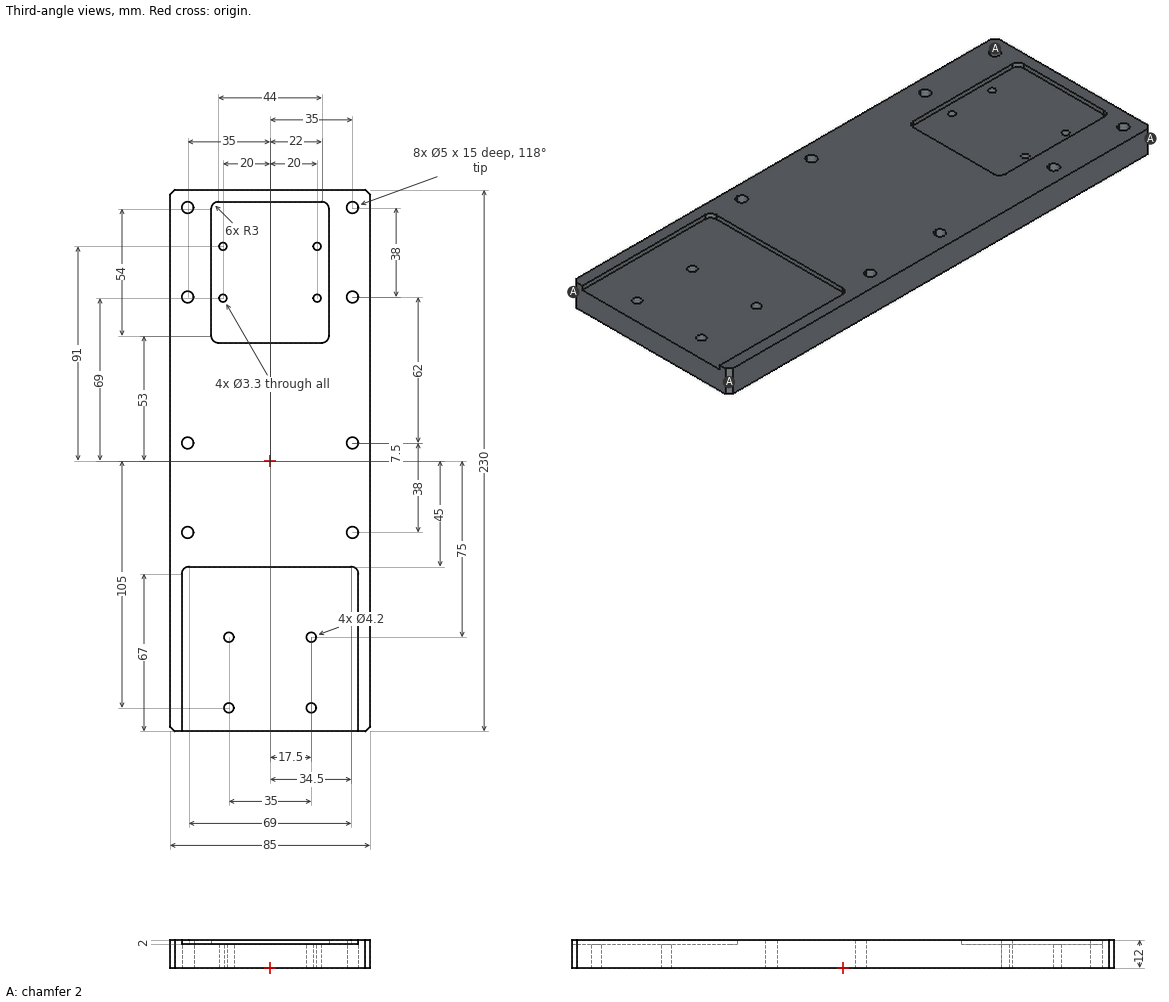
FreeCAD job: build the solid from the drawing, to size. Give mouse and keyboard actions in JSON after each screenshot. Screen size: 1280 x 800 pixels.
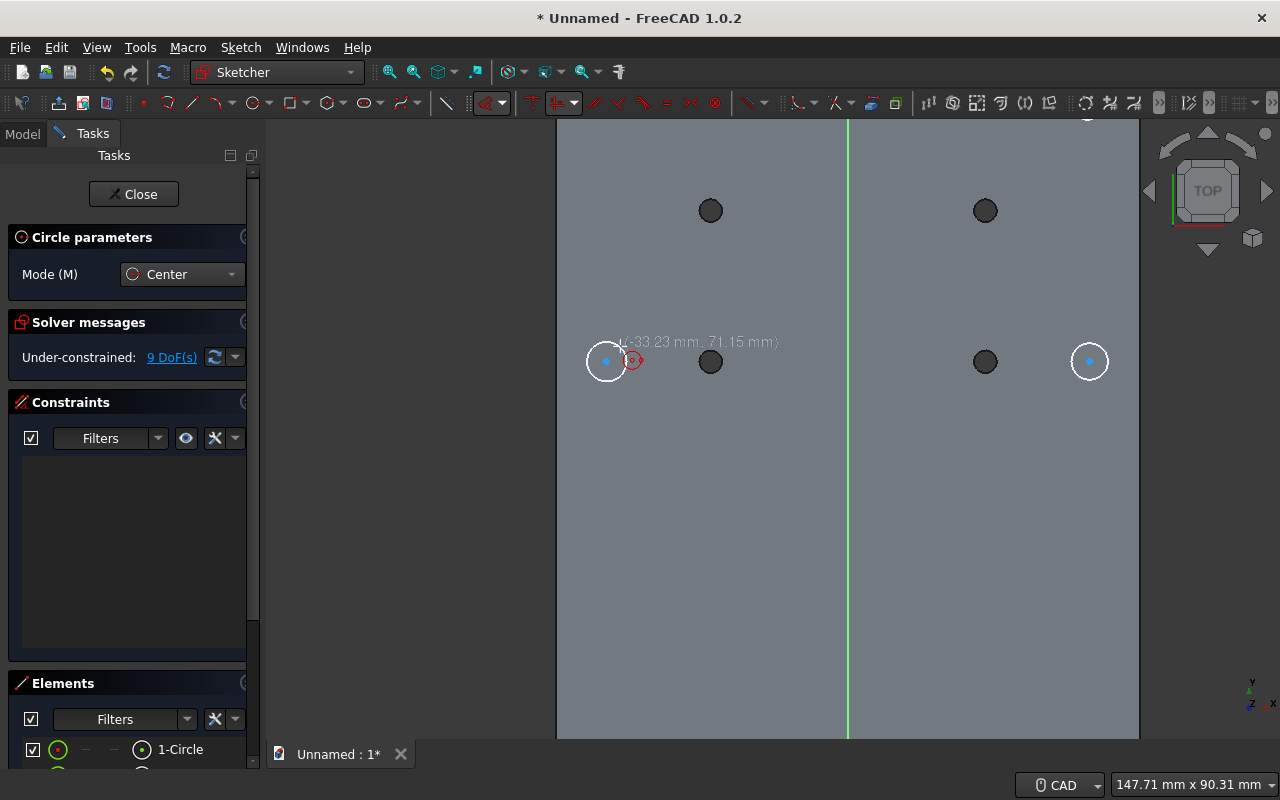
{"action": "scroll", "coordinate": [621, 346], "scroll_direction": "down", "scroll_amount": 5}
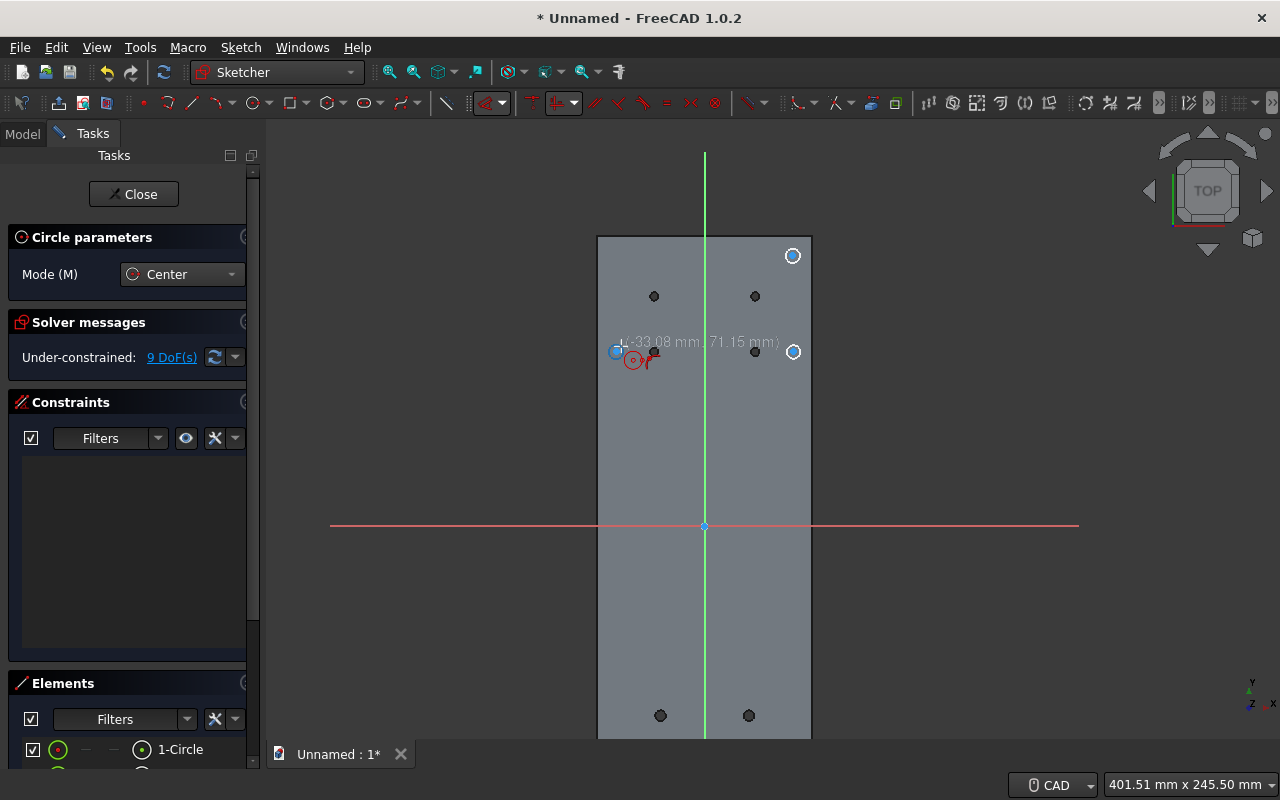
{"action": "scroll", "coordinate": [616, 255], "scroll_direction": "up", "scroll_amount": 7}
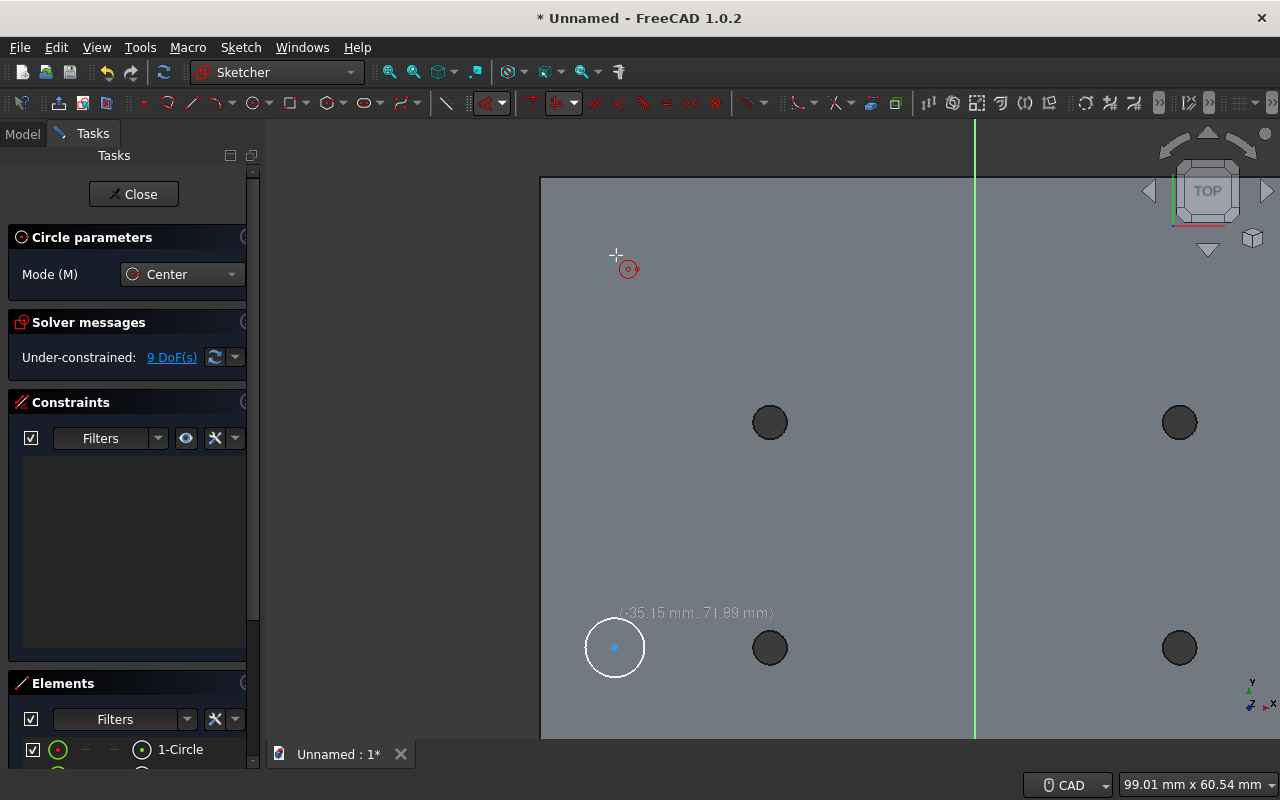
{"action": "scroll", "coordinate": [616, 255], "scroll_direction": "down", "scroll_amount": 7}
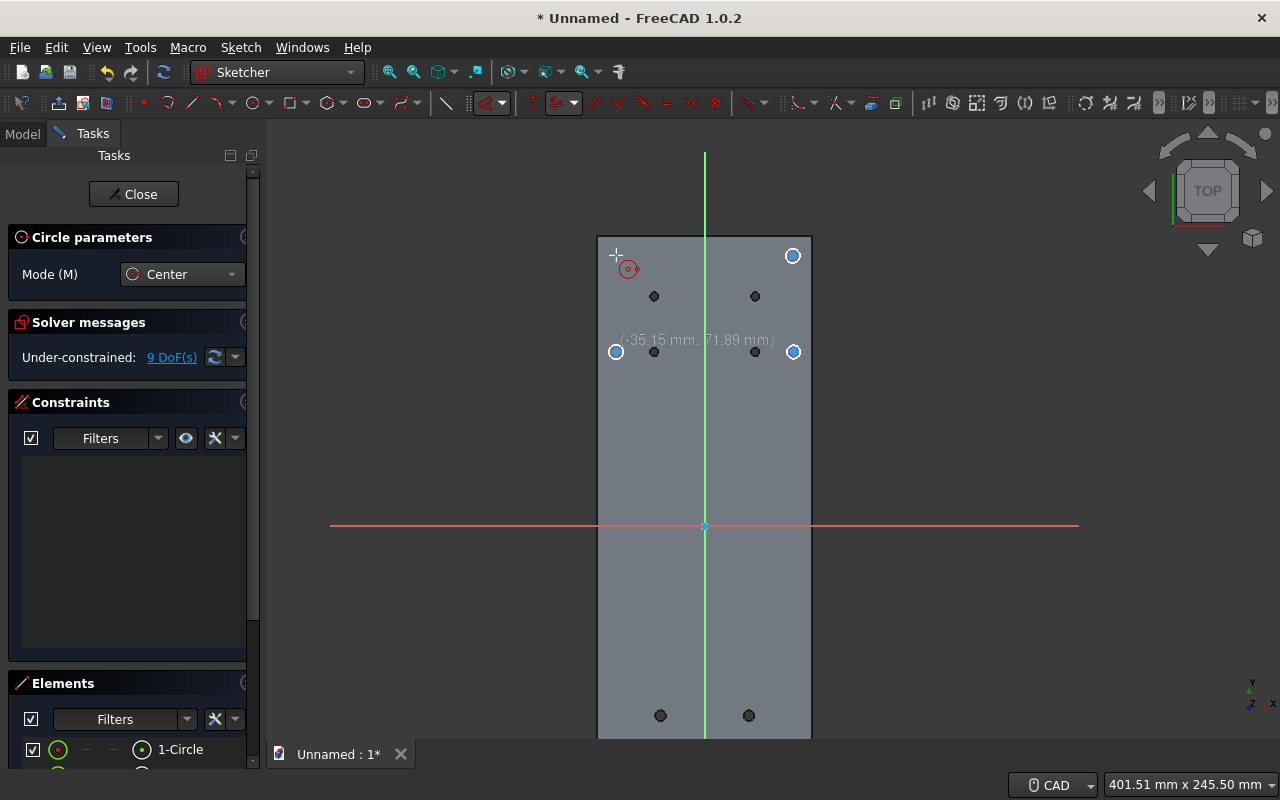
{"action": "left_click", "coordinate": [616, 255]}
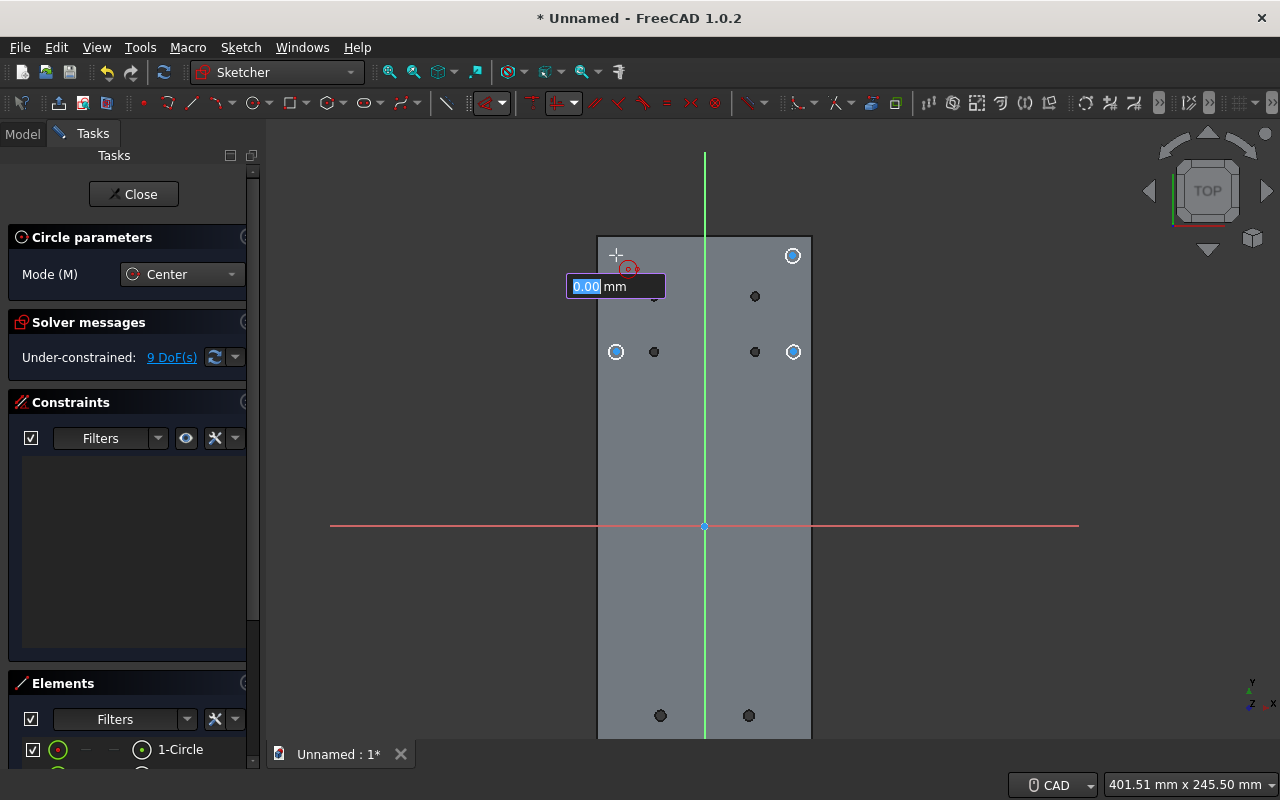
{"action": "scroll", "coordinate": [621, 250], "scroll_direction": "up", "scroll_amount": 5}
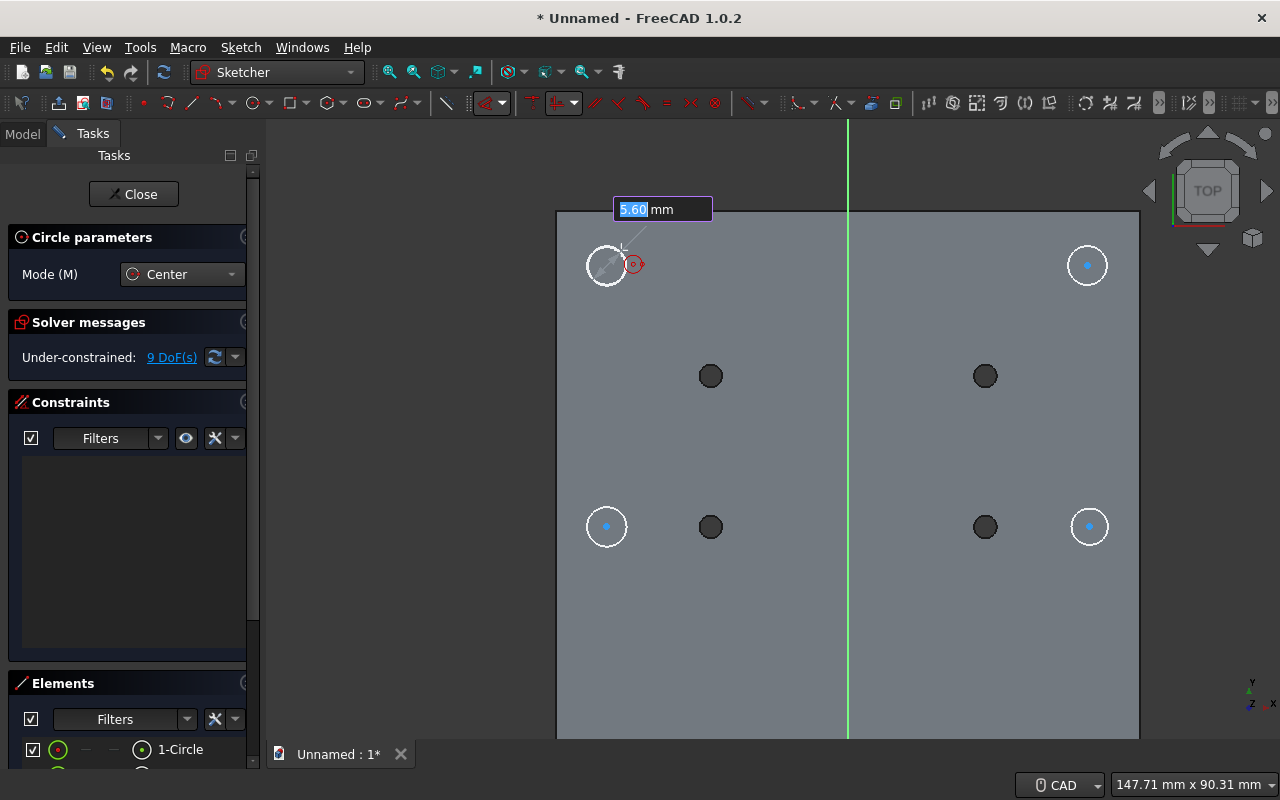
{"action": "left_click", "coordinate": [620, 251]}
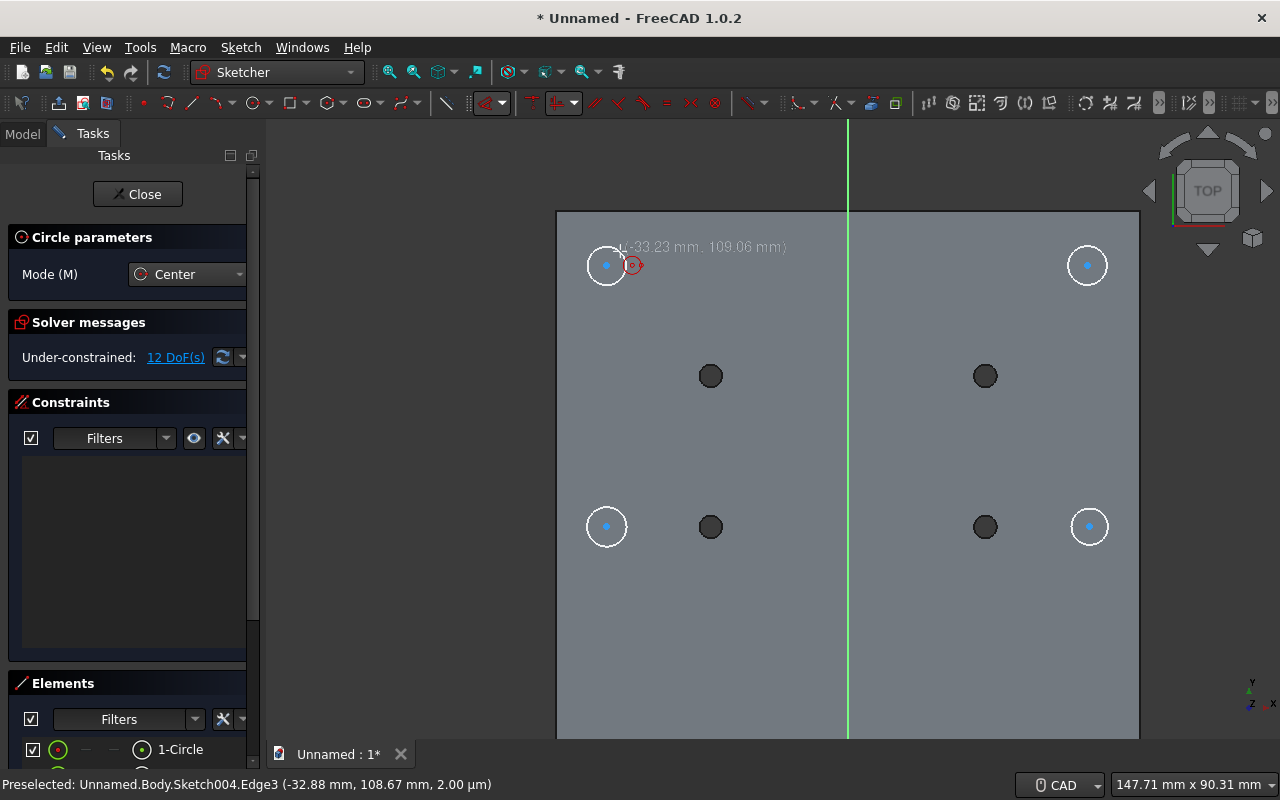
{"action": "scroll", "coordinate": [621, 250], "scroll_direction": "down", "scroll_amount": 5}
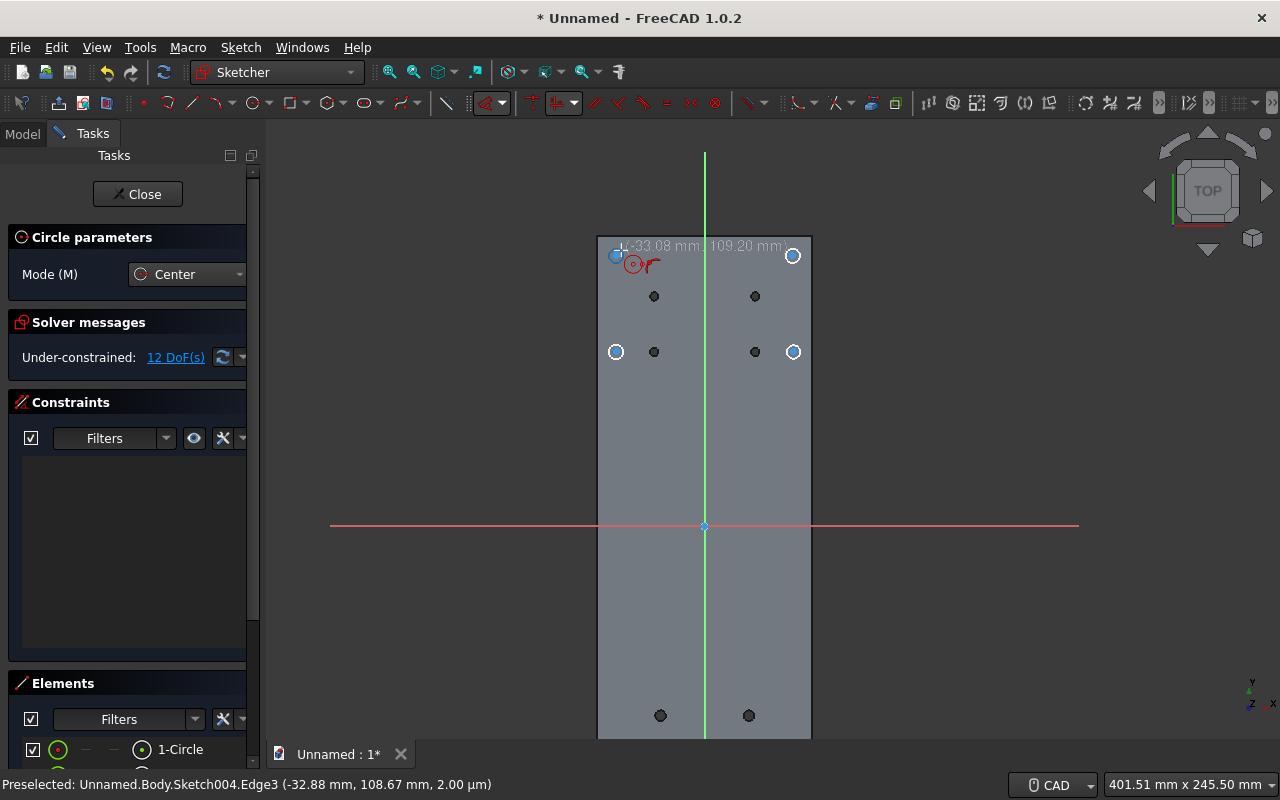
{"action": "scroll", "coordinate": [793, 507], "scroll_direction": "up", "scroll_amount": 7}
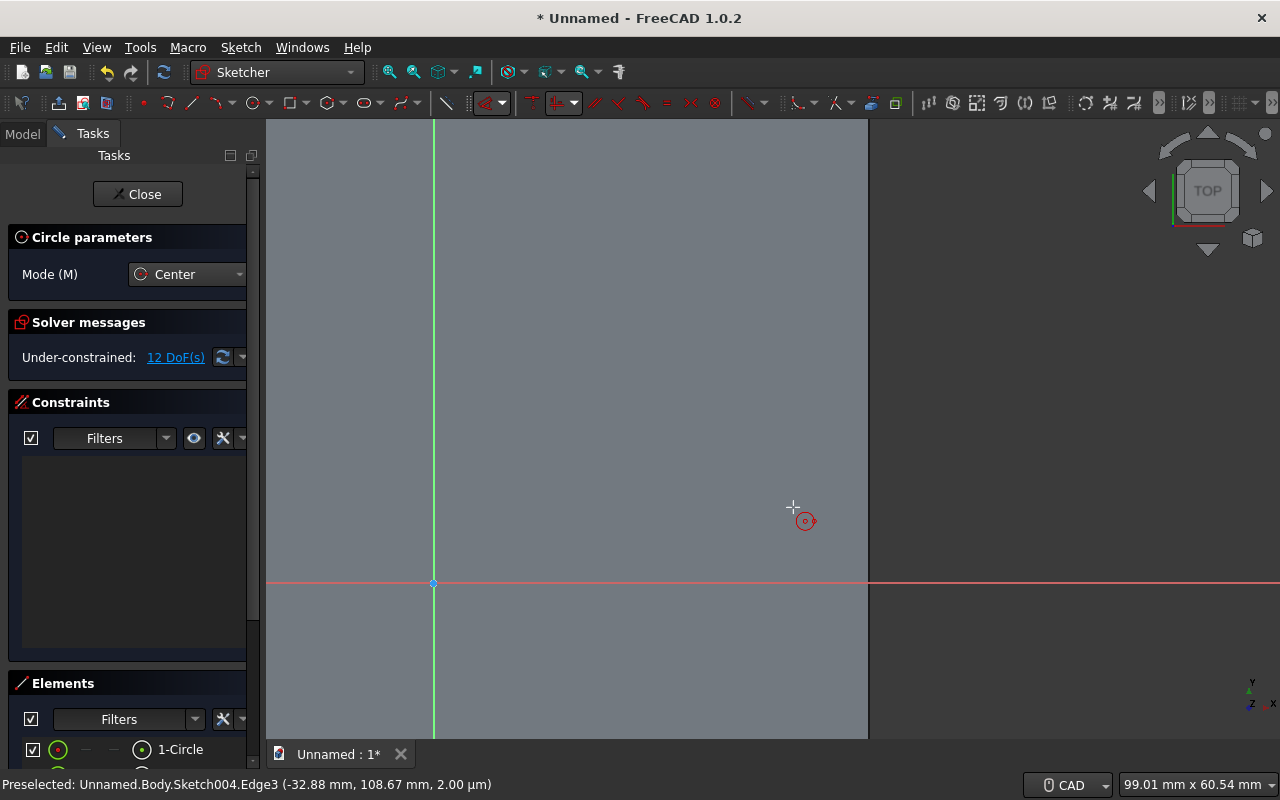
{"action": "scroll", "coordinate": [793, 508], "scroll_direction": "down", "scroll_amount": 7}